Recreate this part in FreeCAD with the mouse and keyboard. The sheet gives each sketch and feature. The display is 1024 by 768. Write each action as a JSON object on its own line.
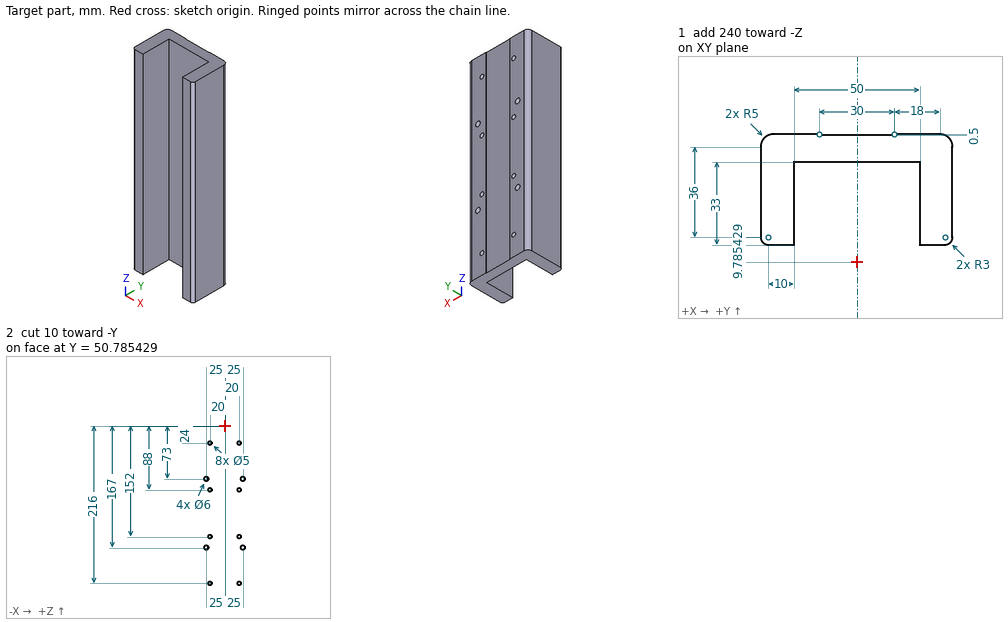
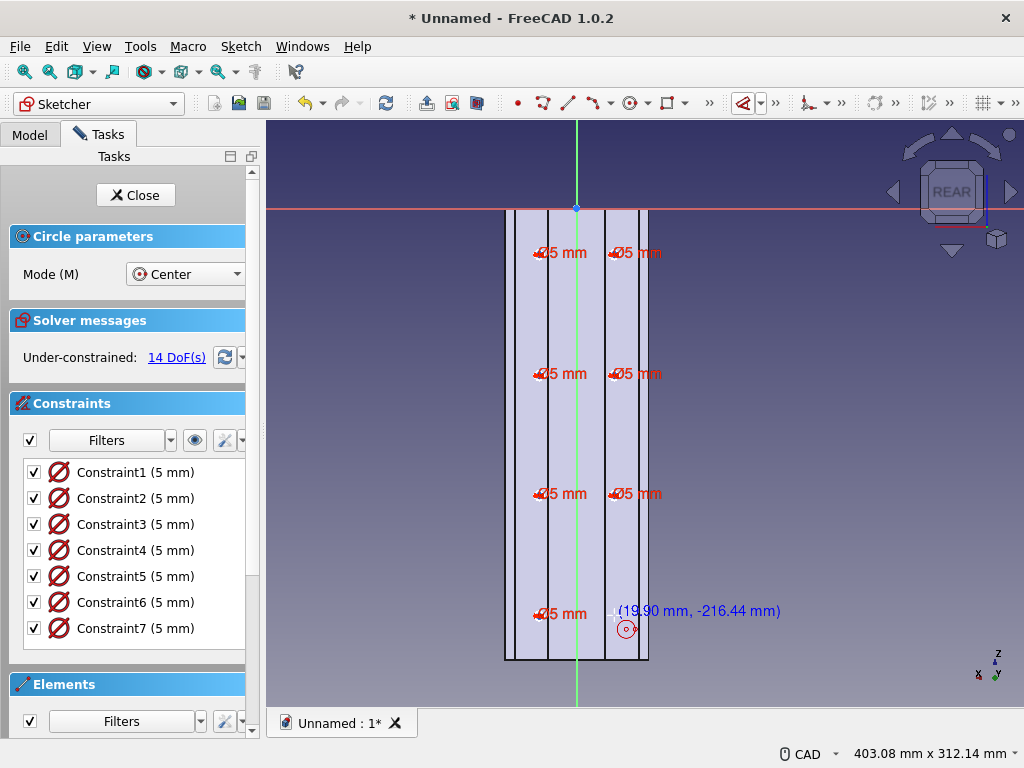
{"action": "left_click", "coordinate": [614, 615]}
{"action": "mouse_move", "coordinate": [618, 612]}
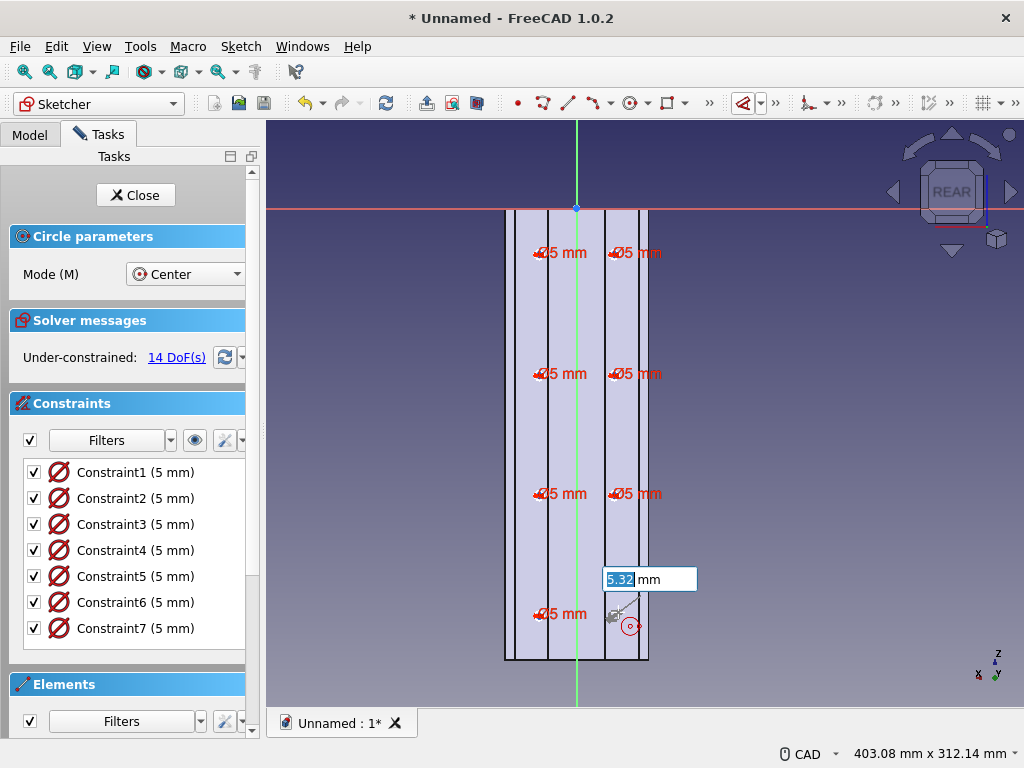
{"action": "type", "text": "5"}
{"action": "key", "text": "Return"}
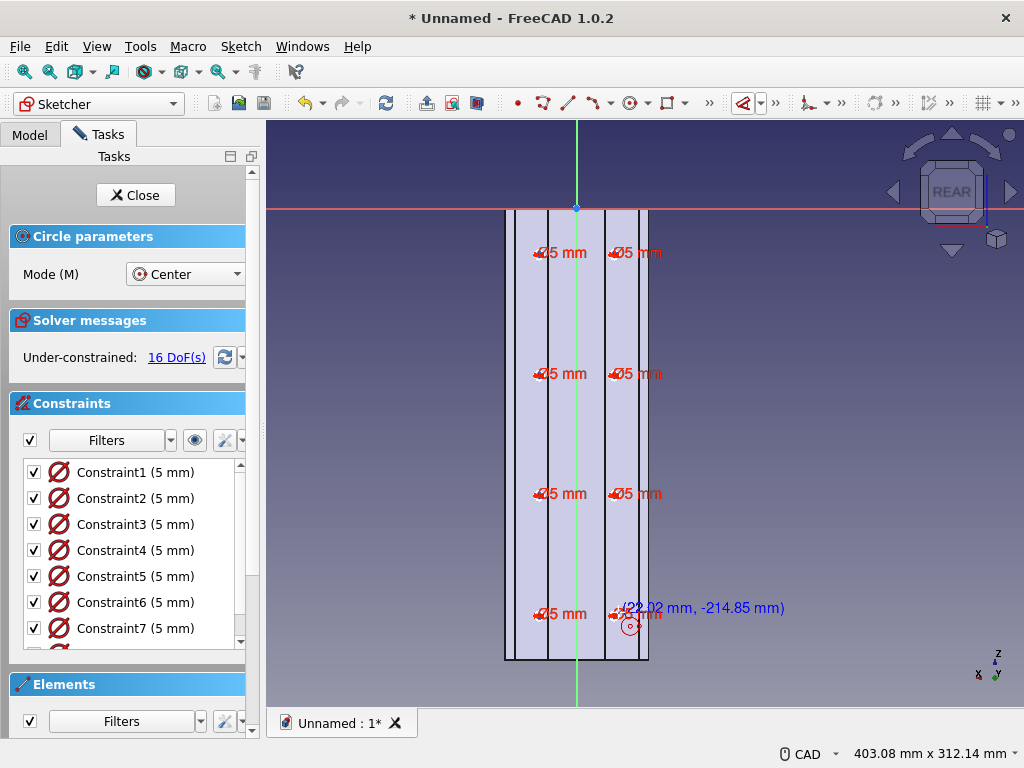
{"action": "scroll", "coordinate": [530, 346], "scroll_direction": "up", "scroll_amount": 7}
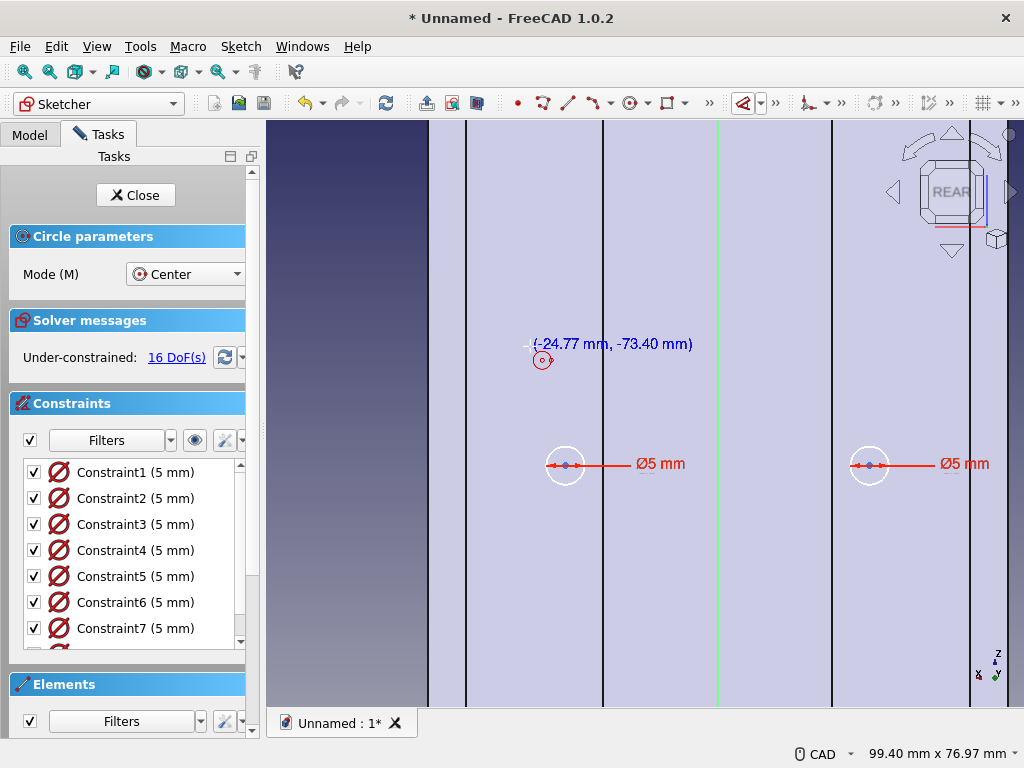
{"action": "scroll", "coordinate": [530, 345], "scroll_direction": "down", "scroll_amount": 7}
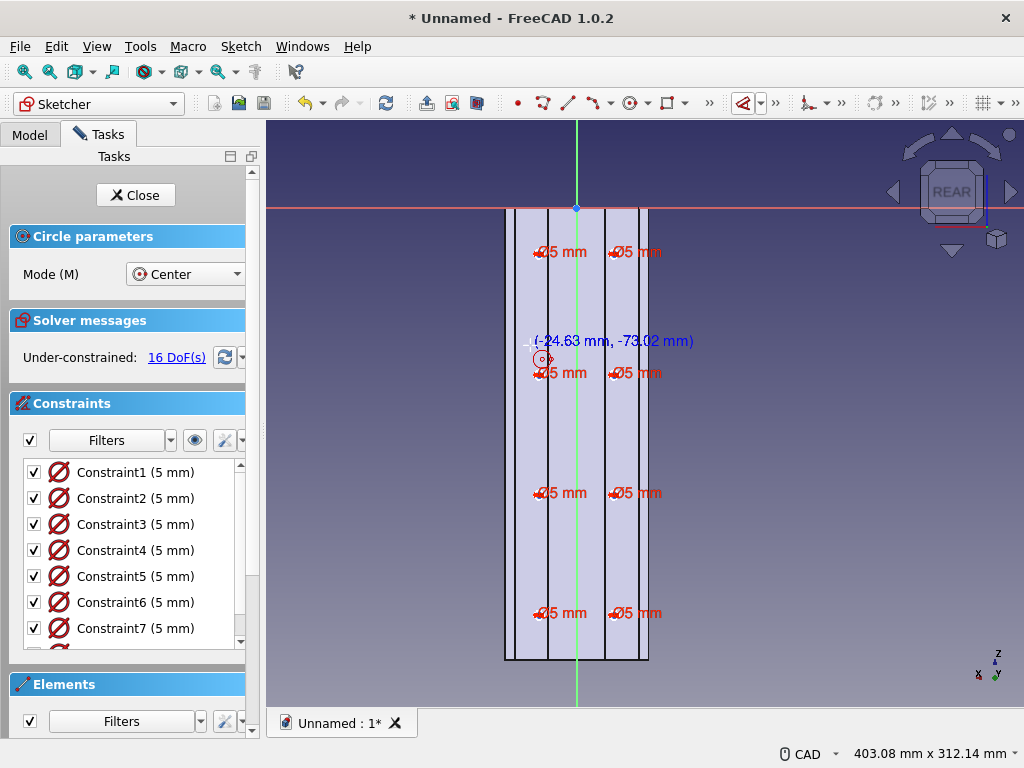
{"action": "left_click", "coordinate": [530, 345]}
{"action": "mouse_move", "coordinate": [534, 342]}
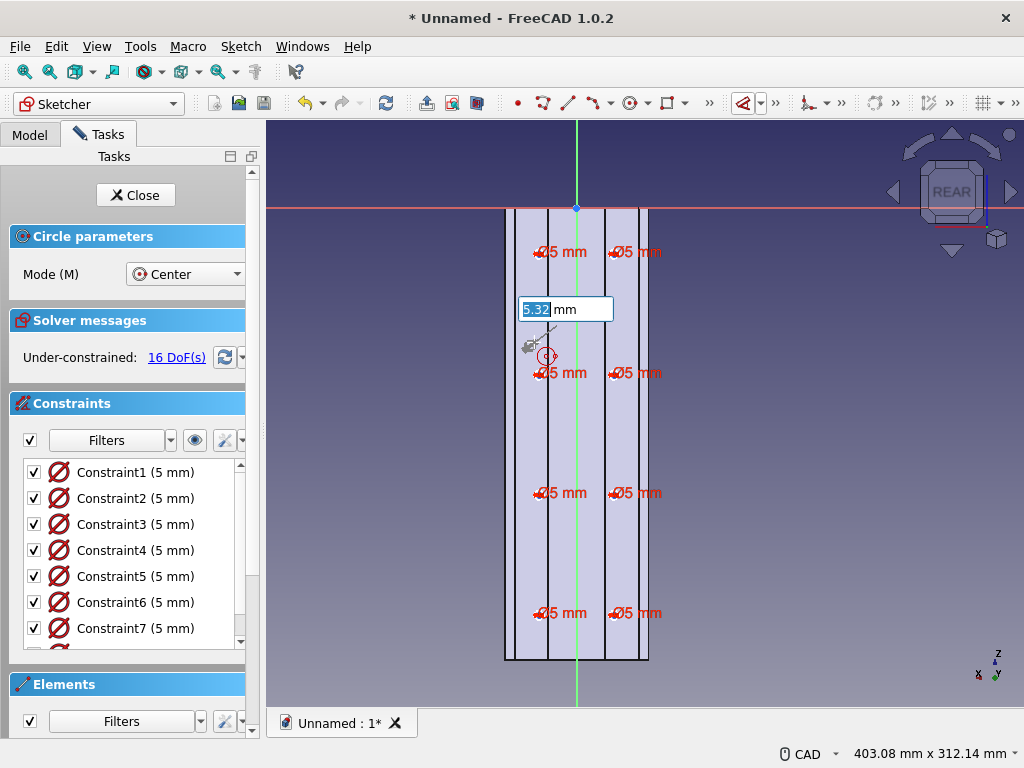
{"action": "type", "text": "6"}
{"action": "key", "text": "Return"}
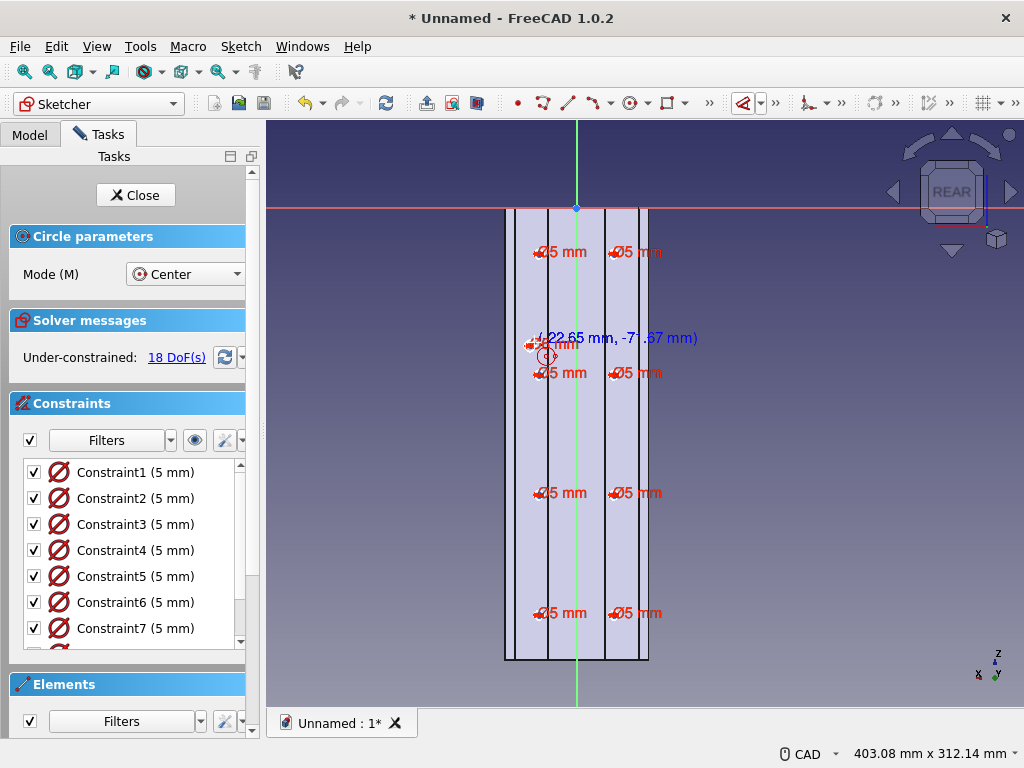
{"action": "scroll", "coordinate": [624, 345], "scroll_direction": "up", "scroll_amount": 7}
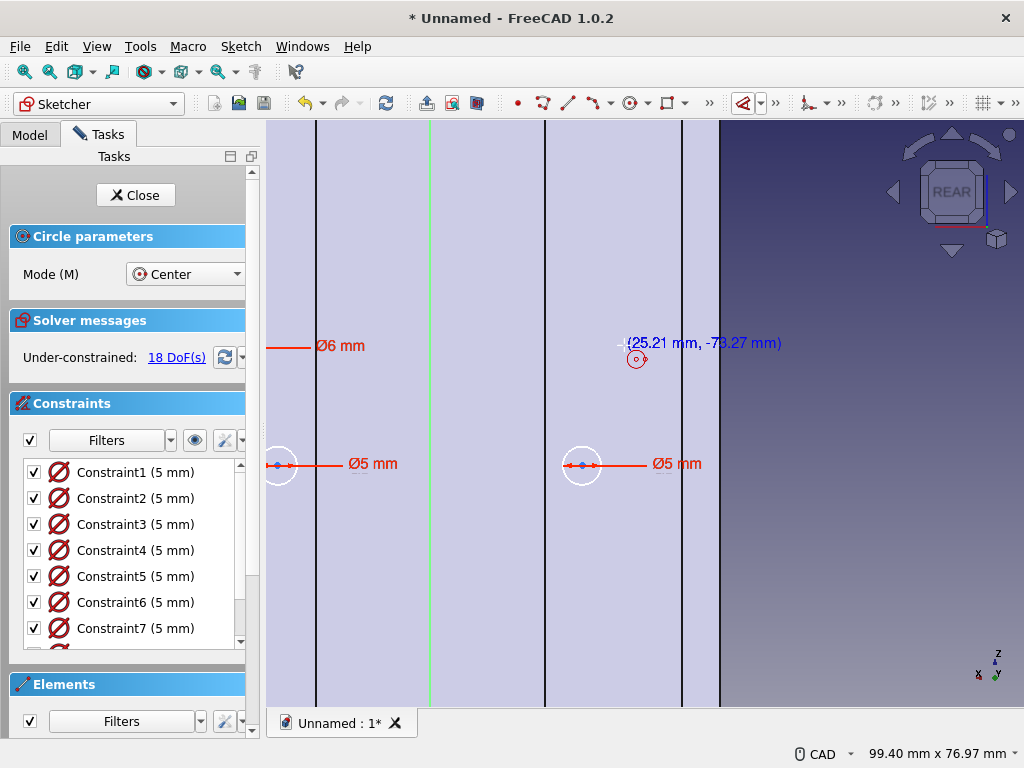
{"action": "scroll", "coordinate": [624, 345], "scroll_direction": "down", "scroll_amount": 7}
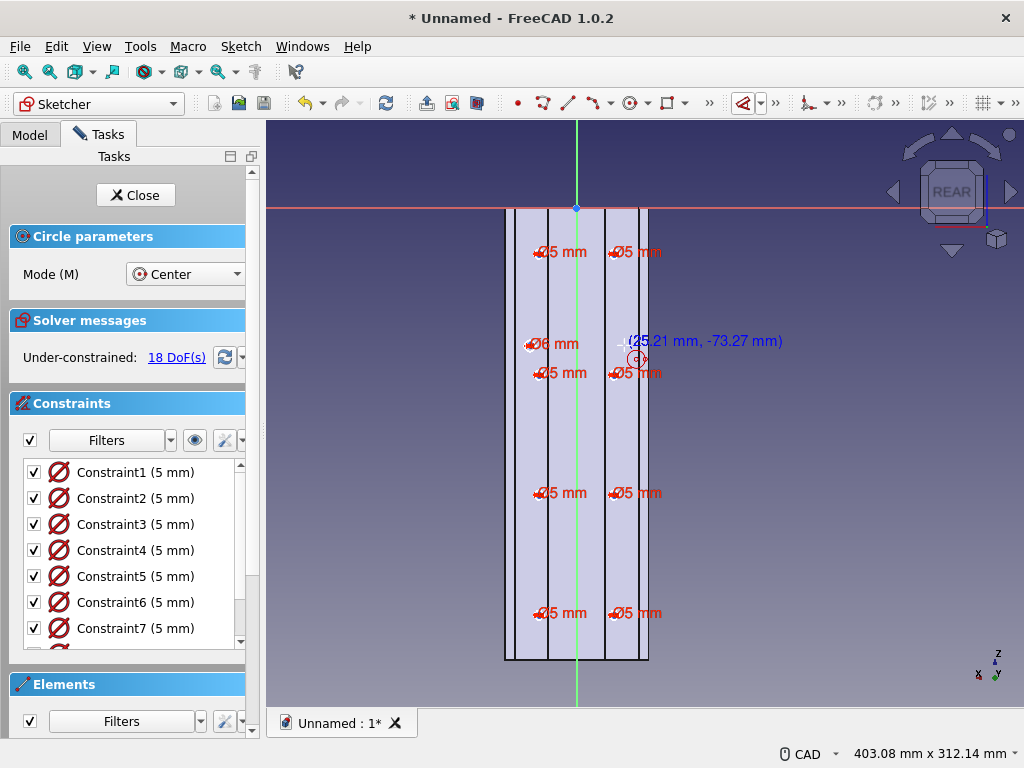
{"action": "left_click", "coordinate": [624, 345]}
{"action": "mouse_move", "coordinate": [628, 342]}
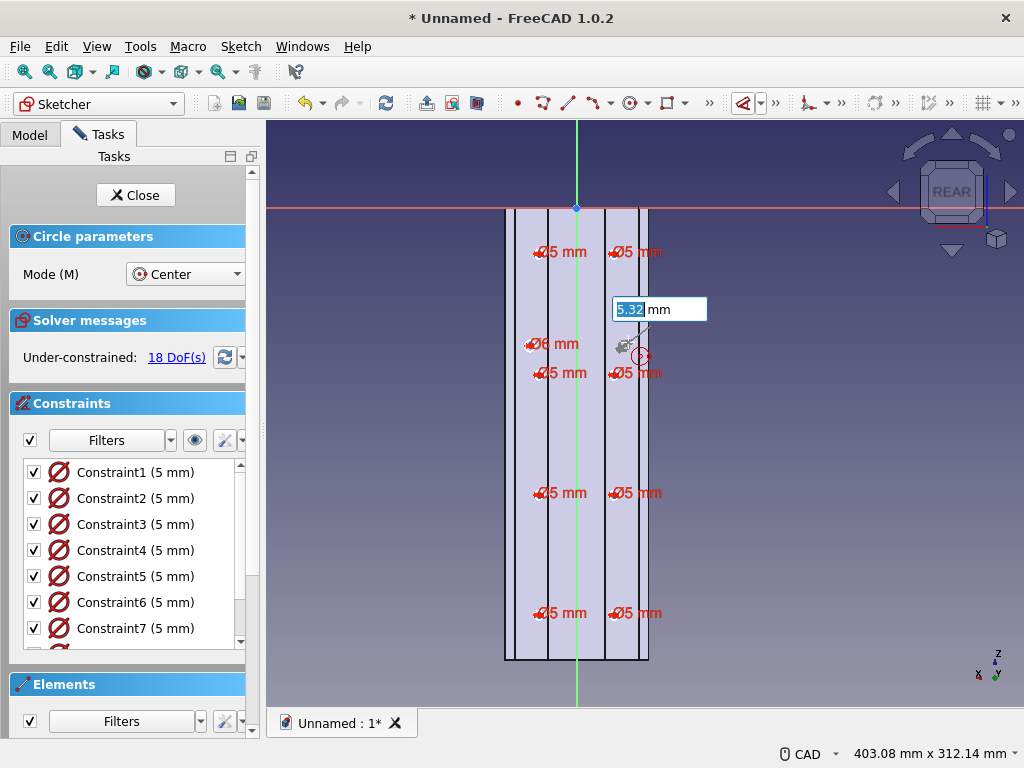
{"action": "type", "text": "6"}
{"action": "key", "text": "Return"}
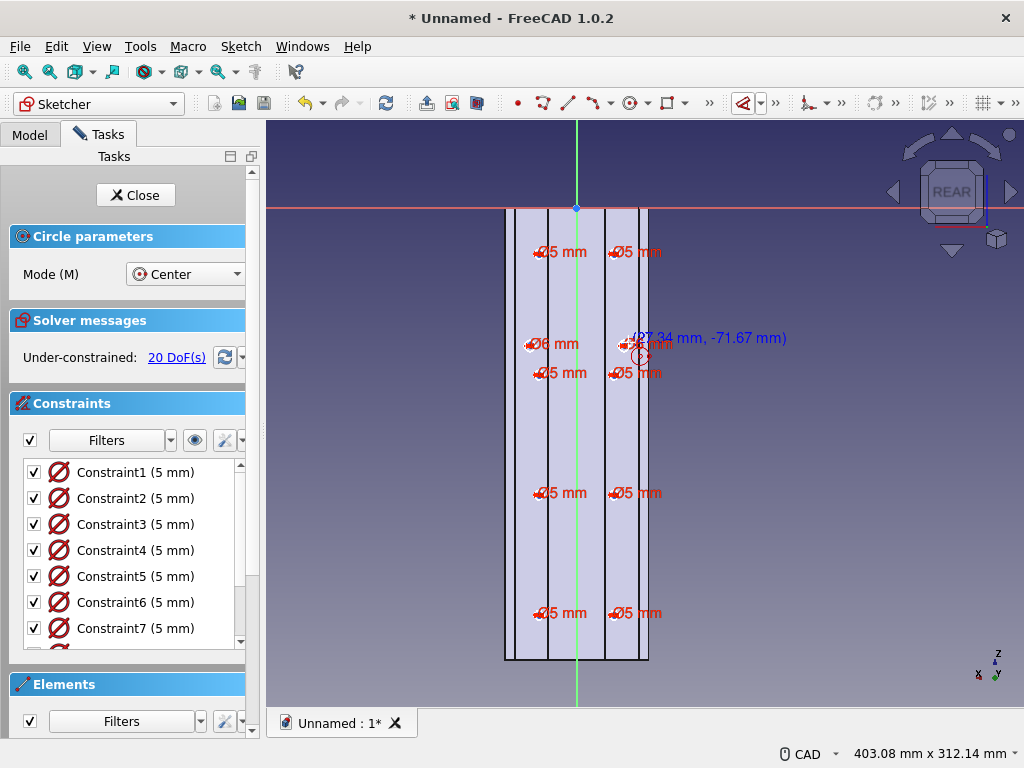
{"action": "scroll", "coordinate": [530, 522], "scroll_direction": "up", "scroll_amount": 7}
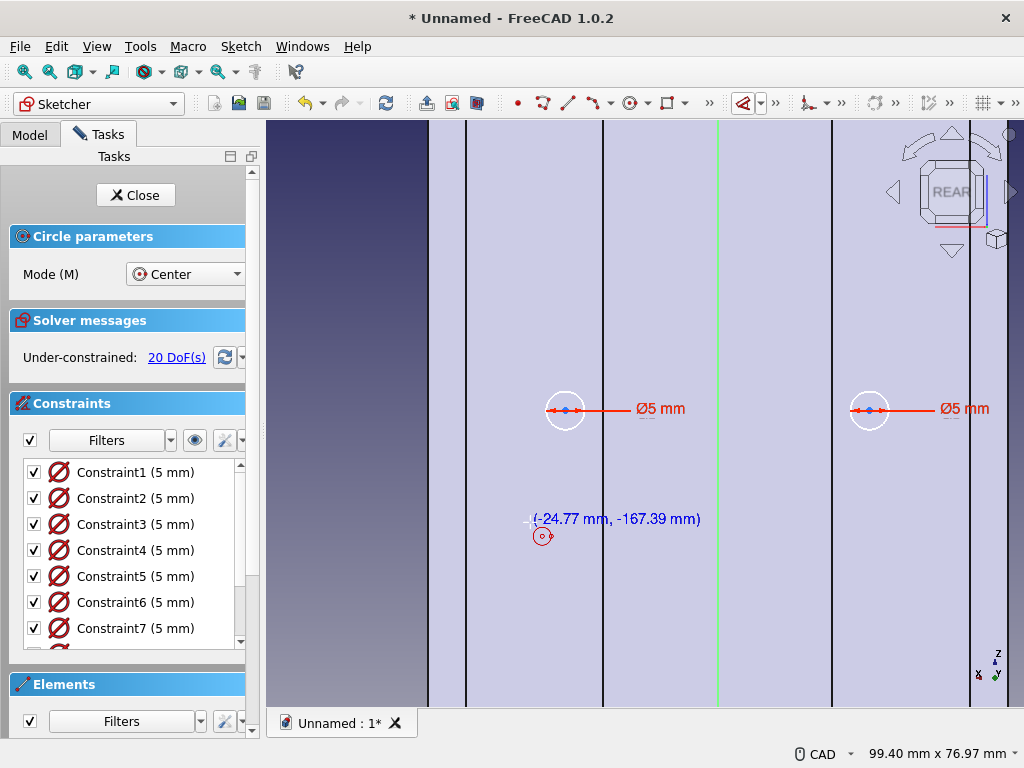
{"action": "scroll", "coordinate": [530, 522], "scroll_direction": "down", "scroll_amount": 7}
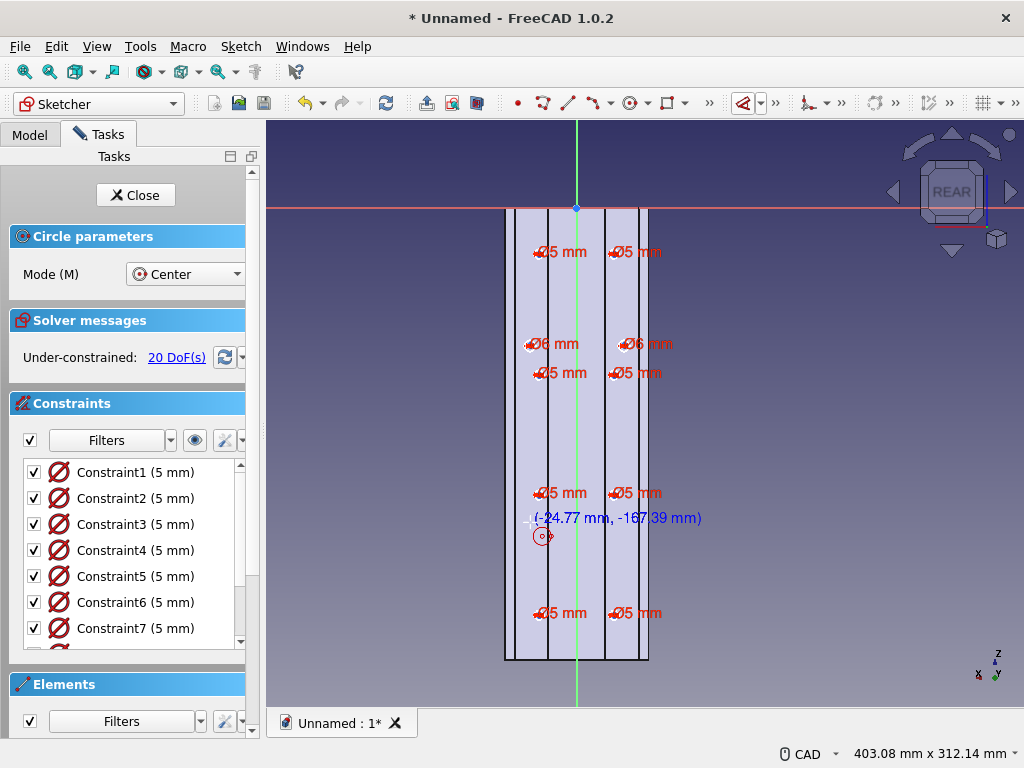
{"action": "left_click", "coordinate": [530, 522]}
{"action": "mouse_move", "coordinate": [534, 518]}